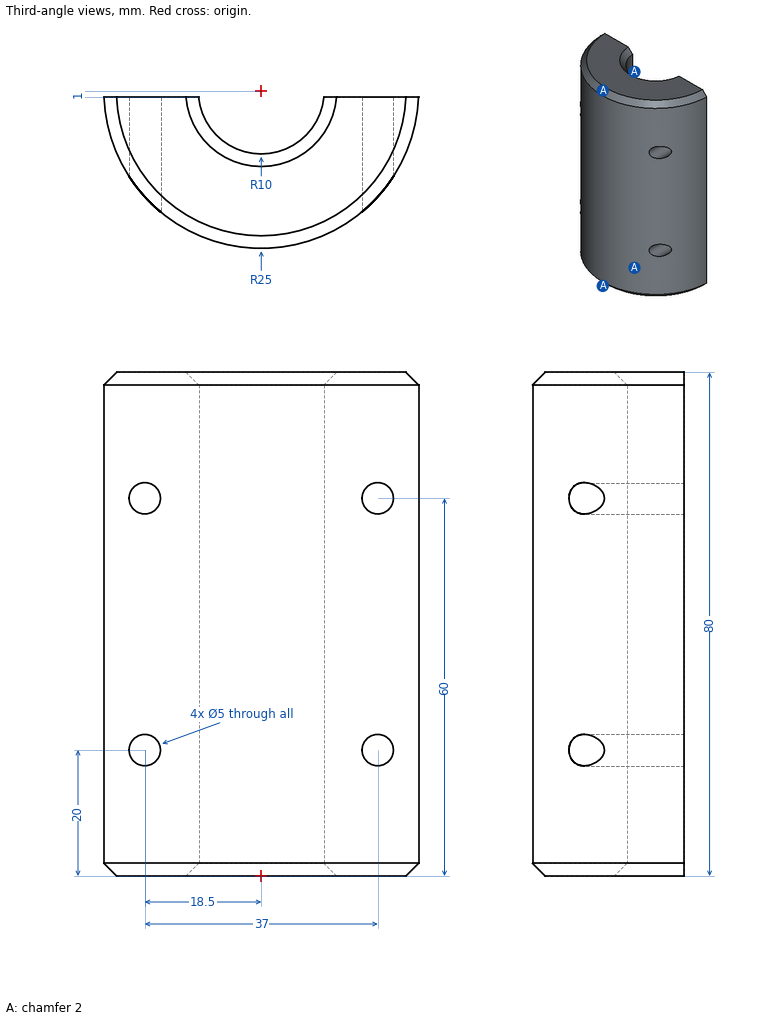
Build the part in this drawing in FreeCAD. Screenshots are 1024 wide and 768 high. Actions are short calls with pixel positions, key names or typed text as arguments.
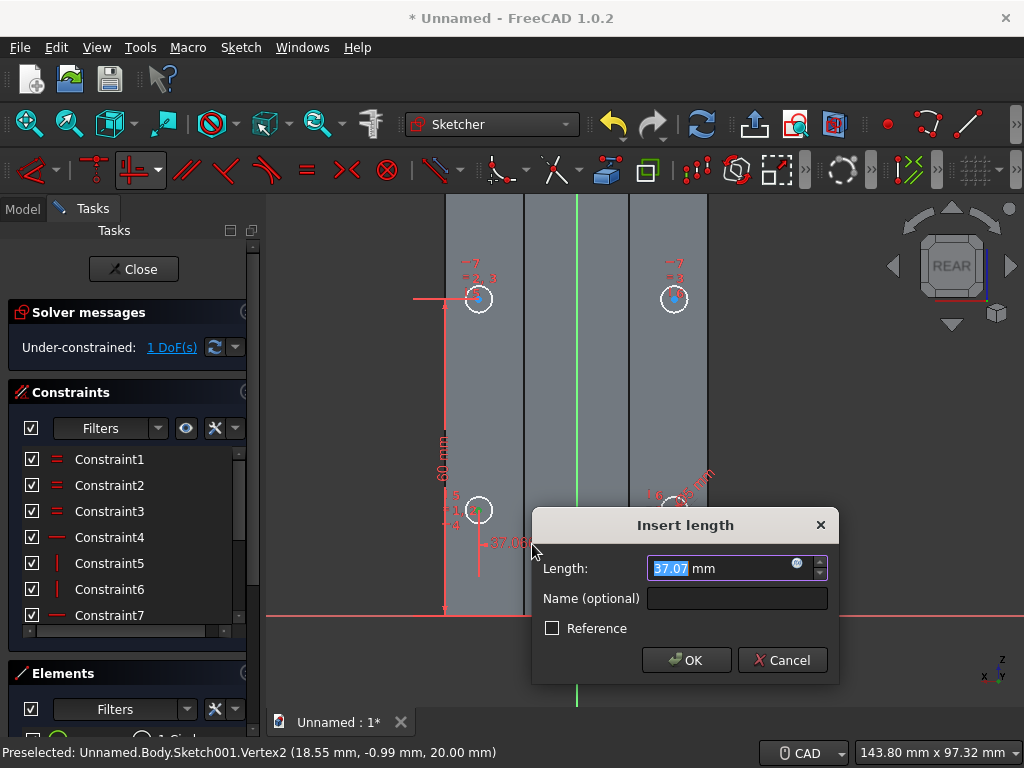
text(37)
key(Return)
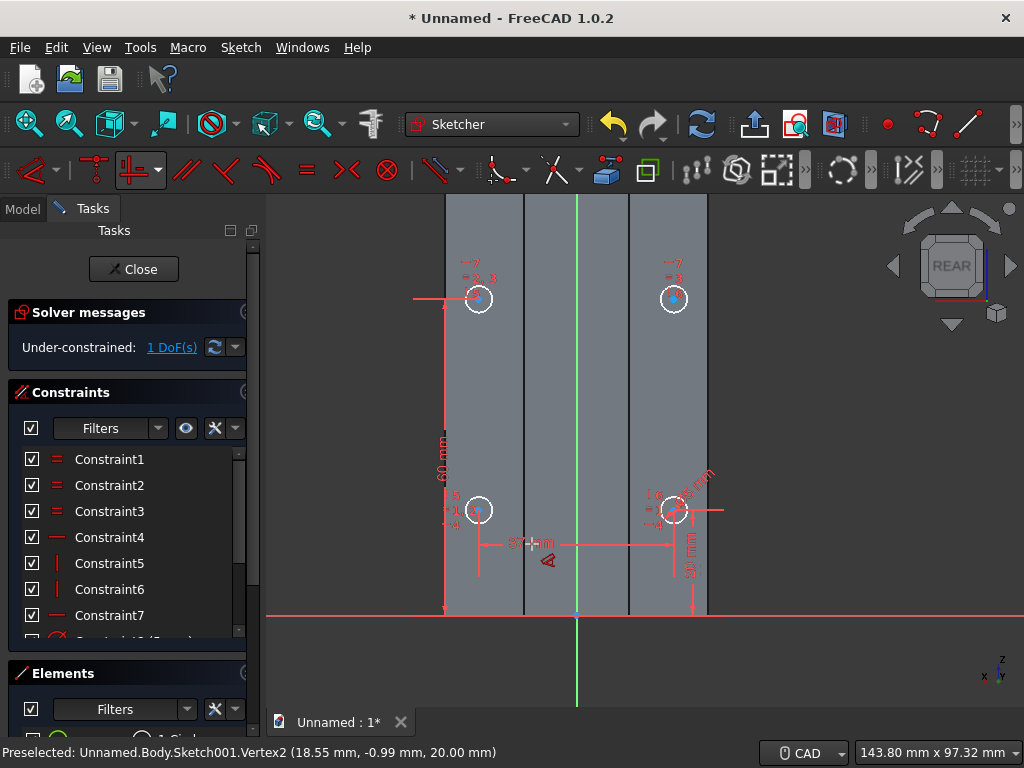
click(674, 510)
click(625, 650)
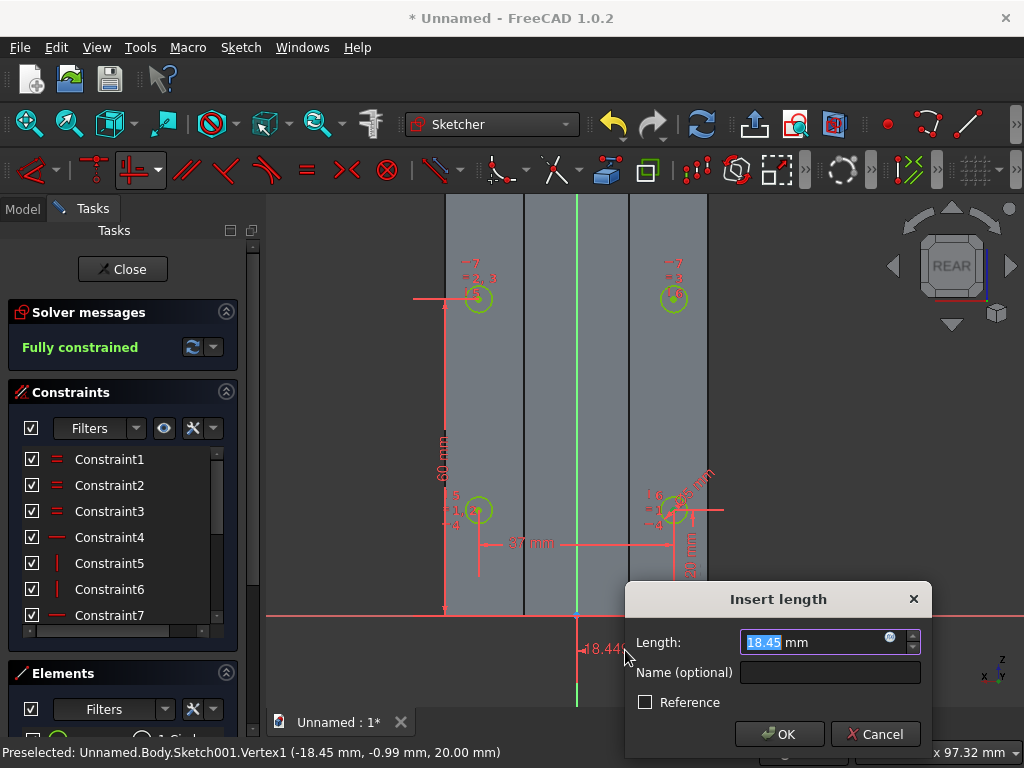
text(18.5)
key(Return)
key(Escape)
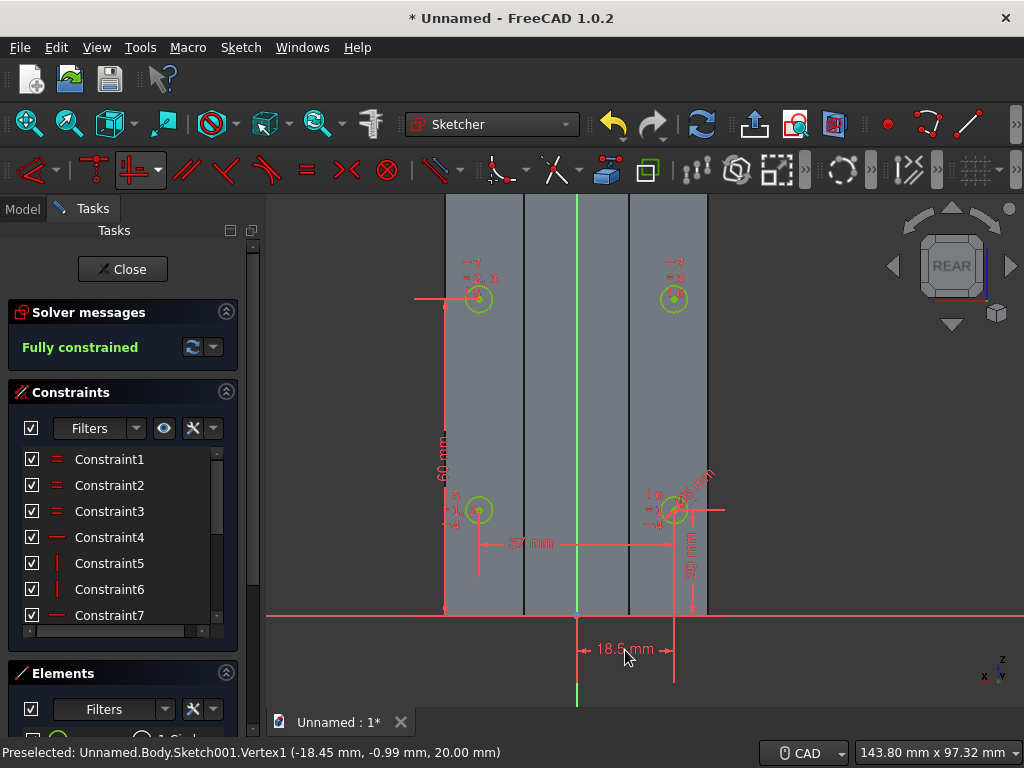
click(123, 269)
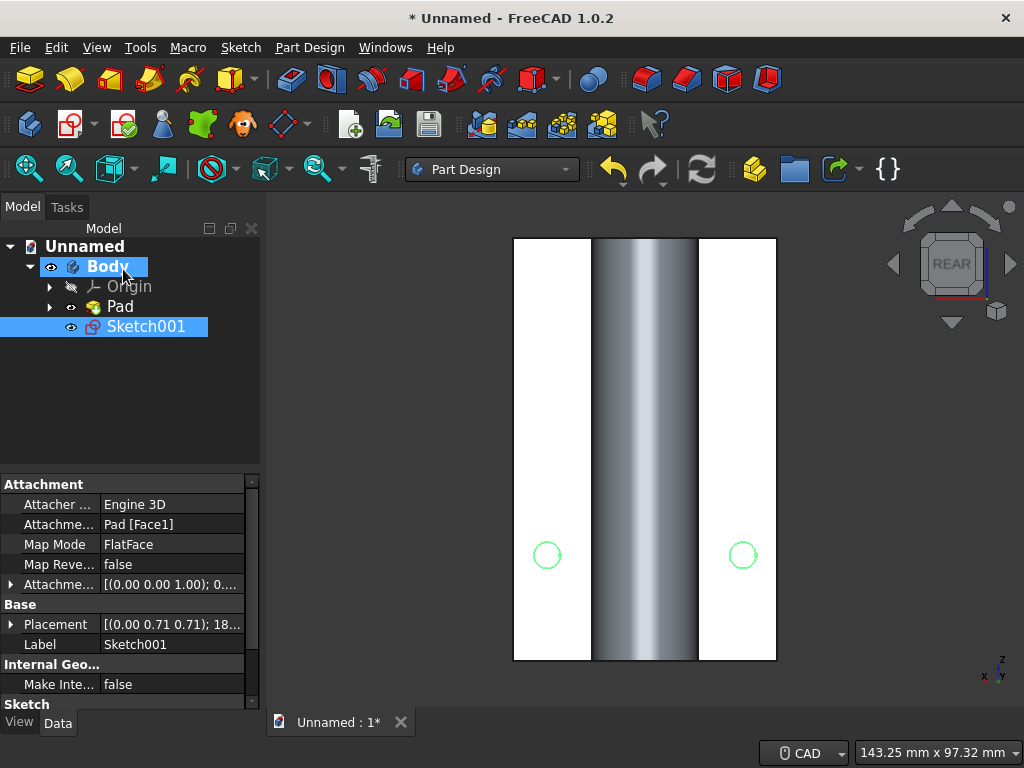
click(332, 80)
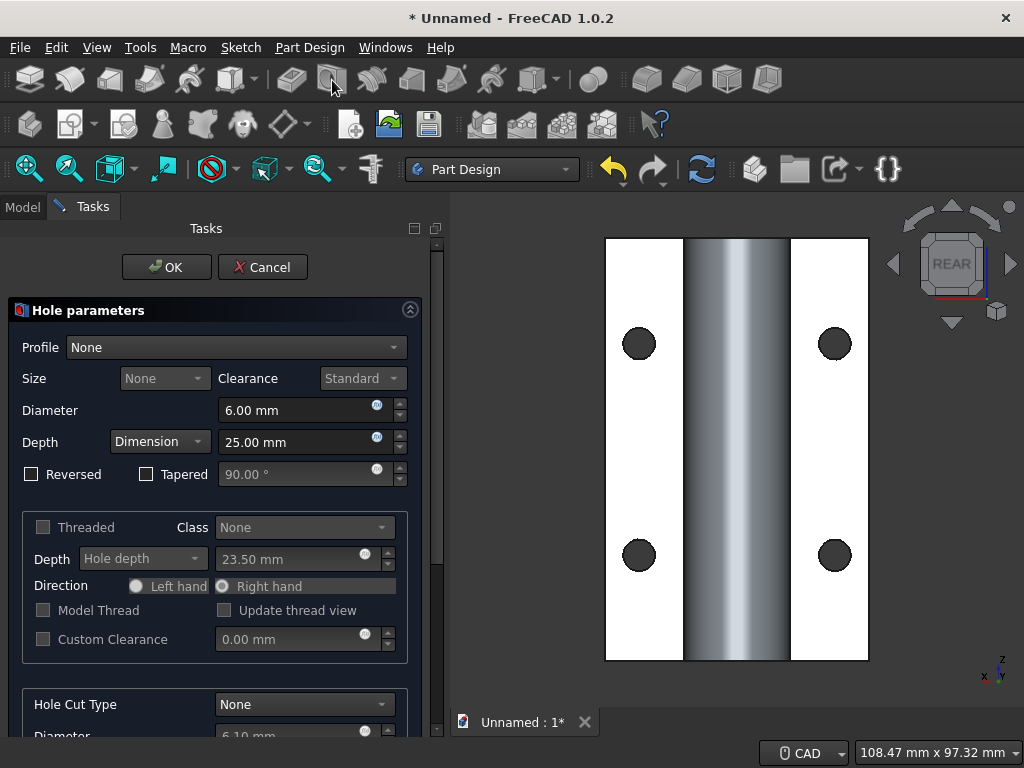
triple_click(305, 410)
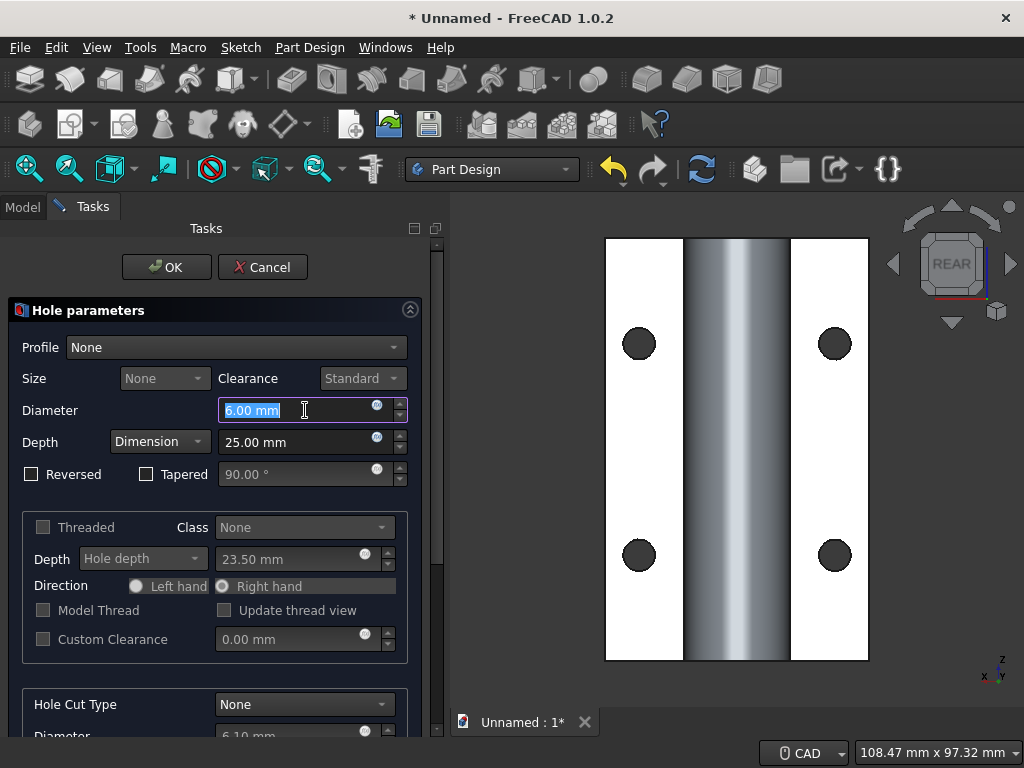
text(5)
key(Tab)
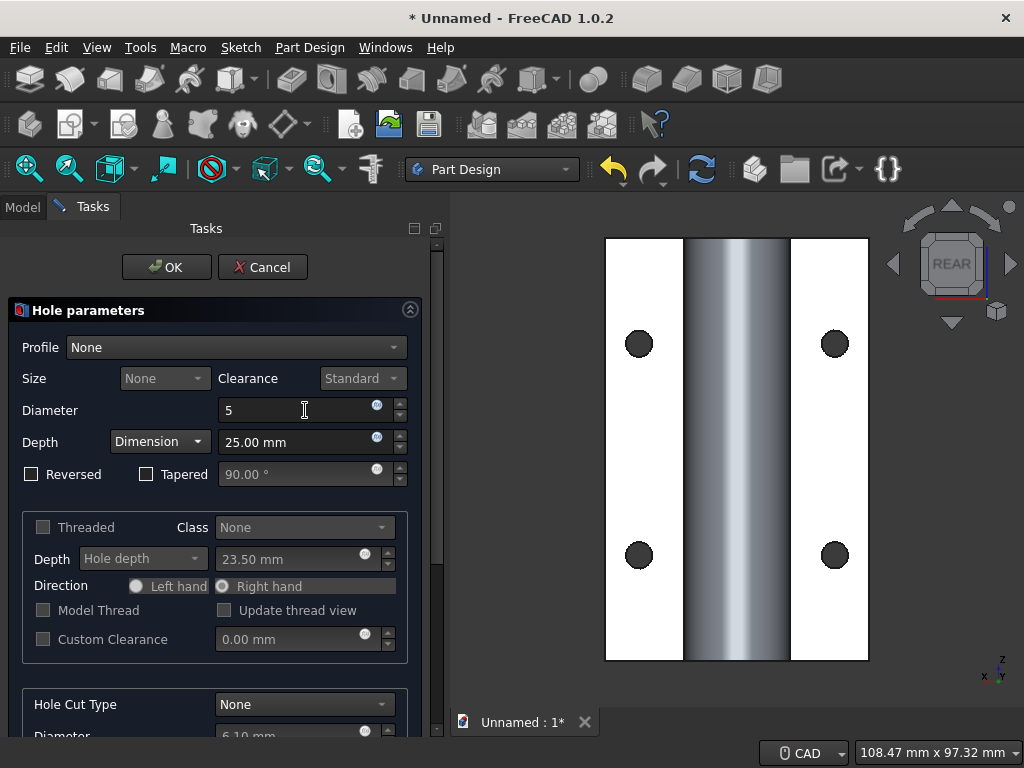
click(161, 442)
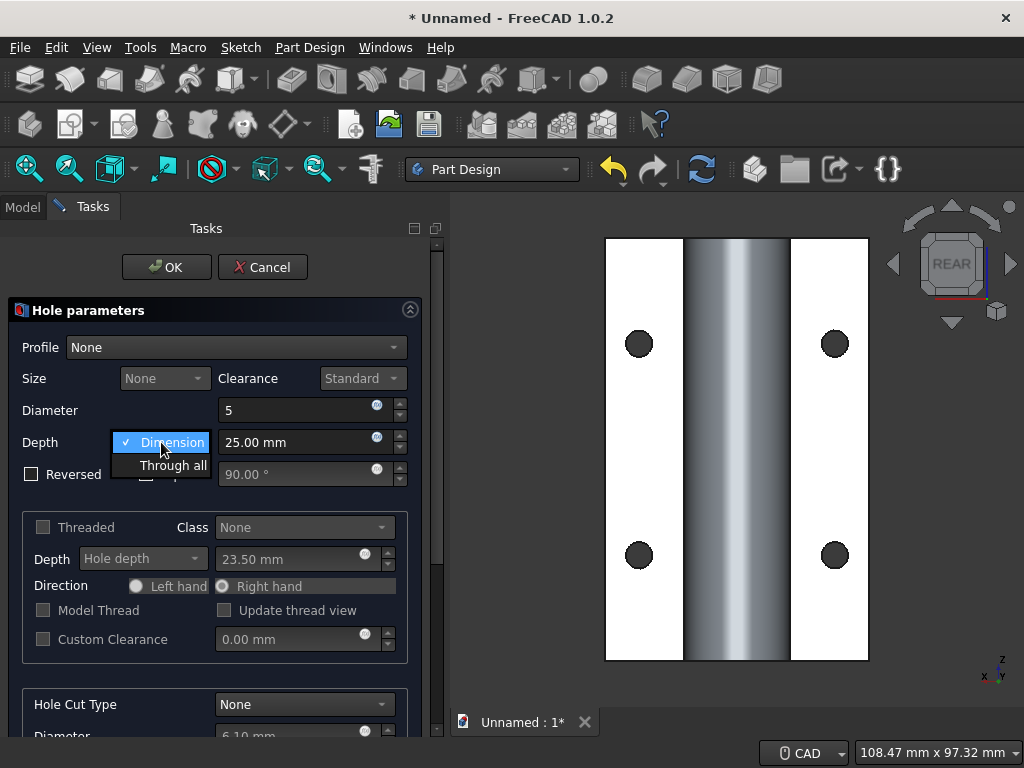
click(160, 466)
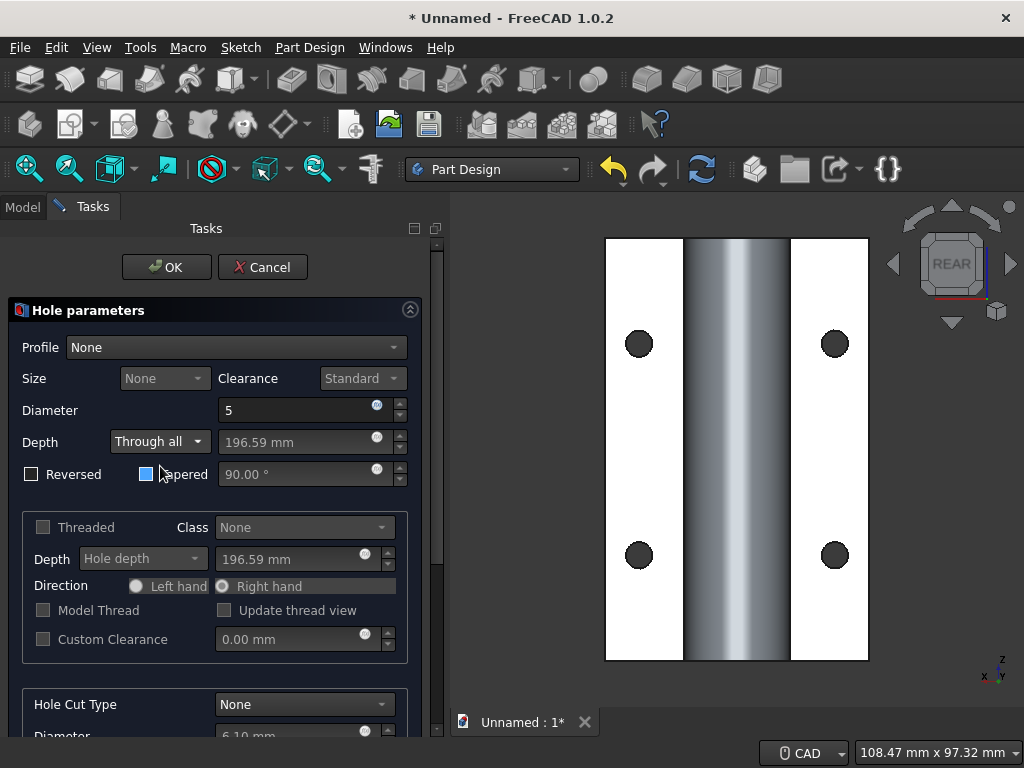
click(167, 267)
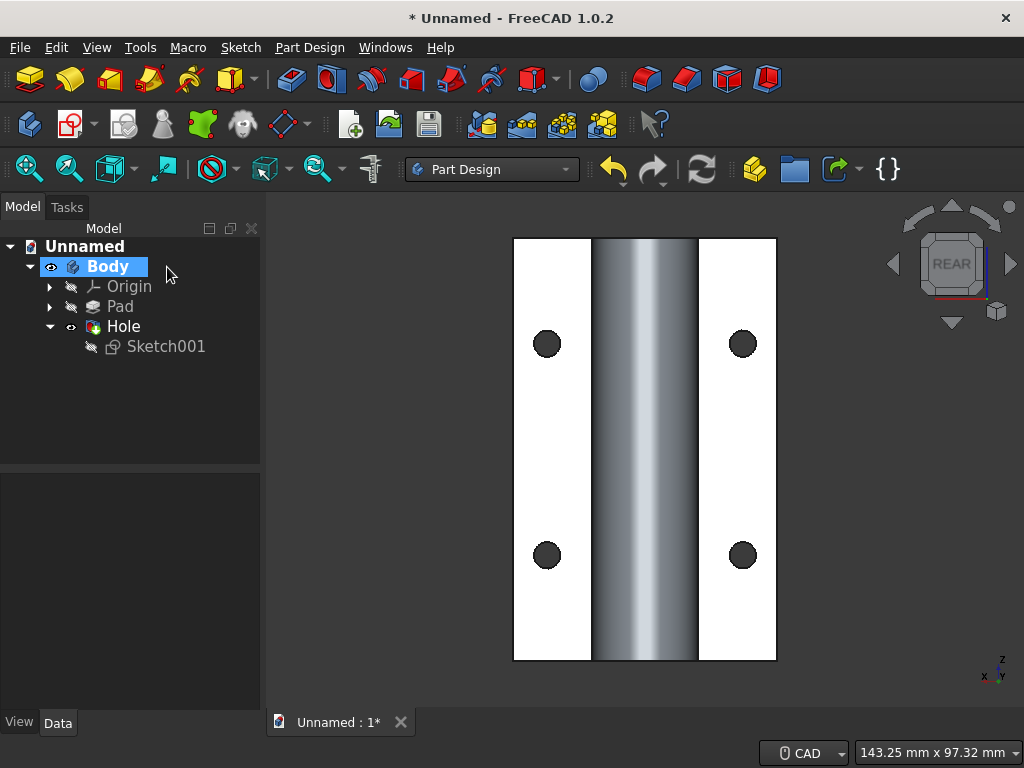
click(645, 237)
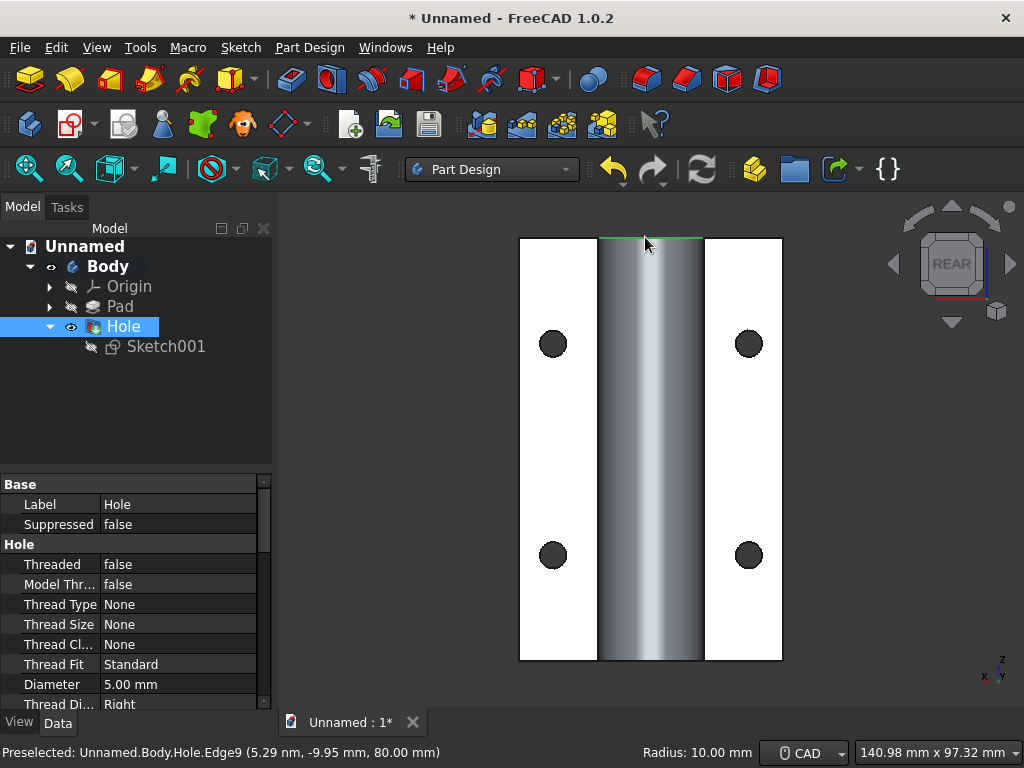
click(651, 660, ctrl)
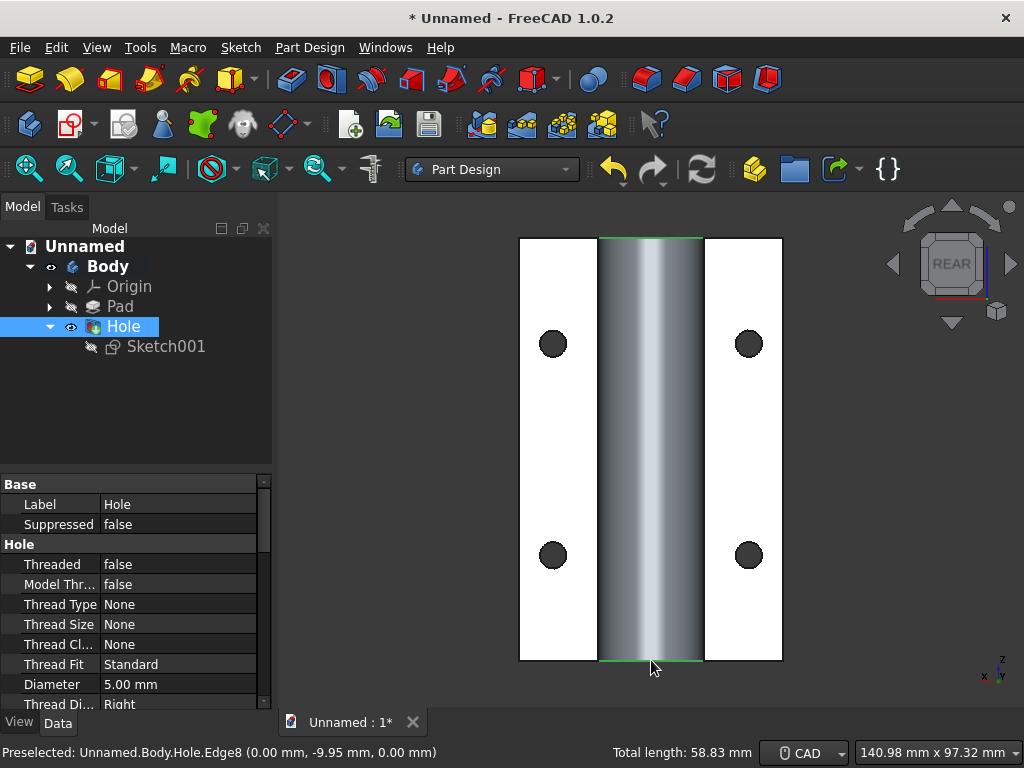
key(0)